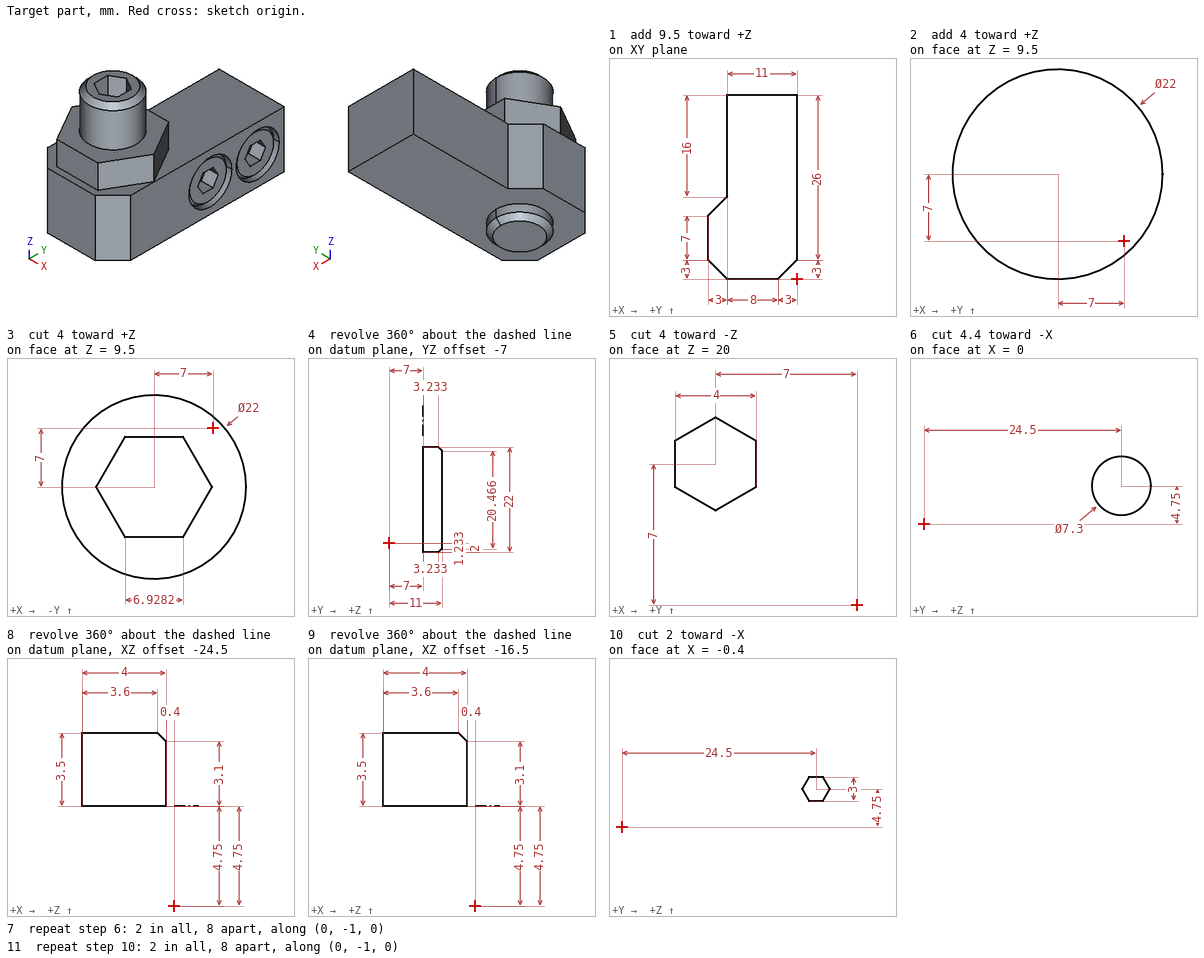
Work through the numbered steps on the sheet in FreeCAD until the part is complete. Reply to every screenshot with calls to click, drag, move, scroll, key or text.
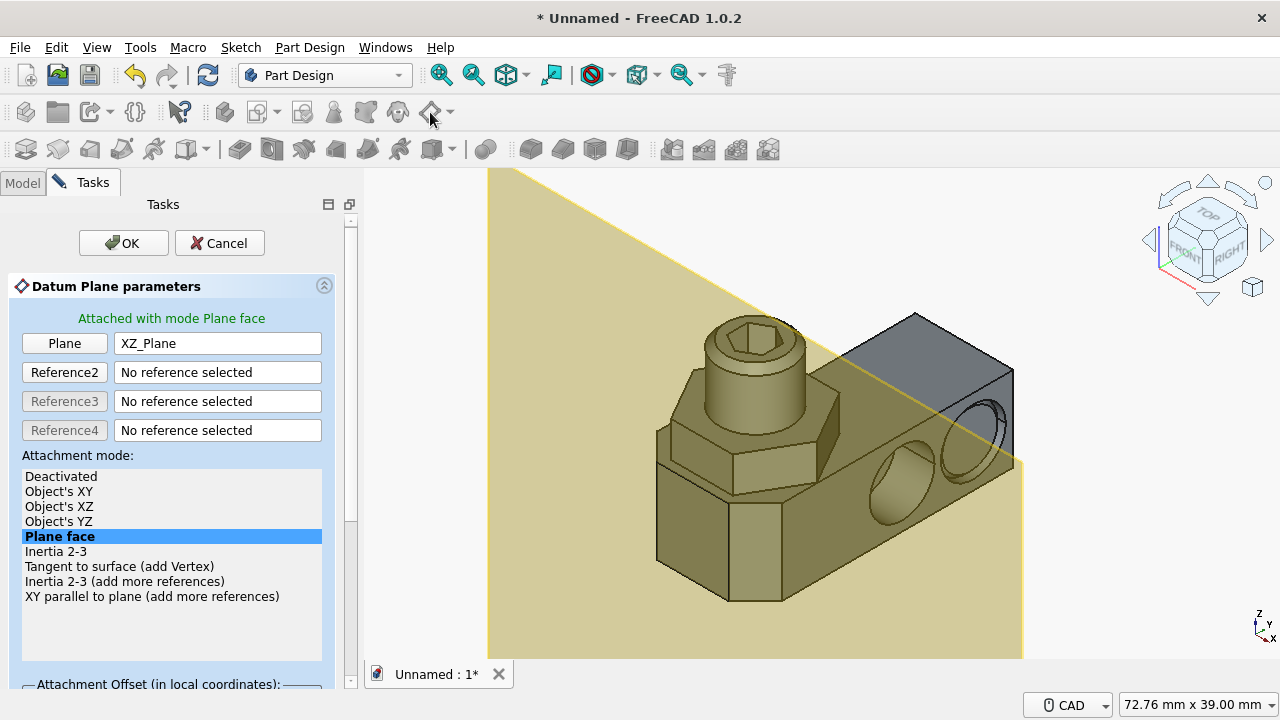
scroll(351, 451, down, 3)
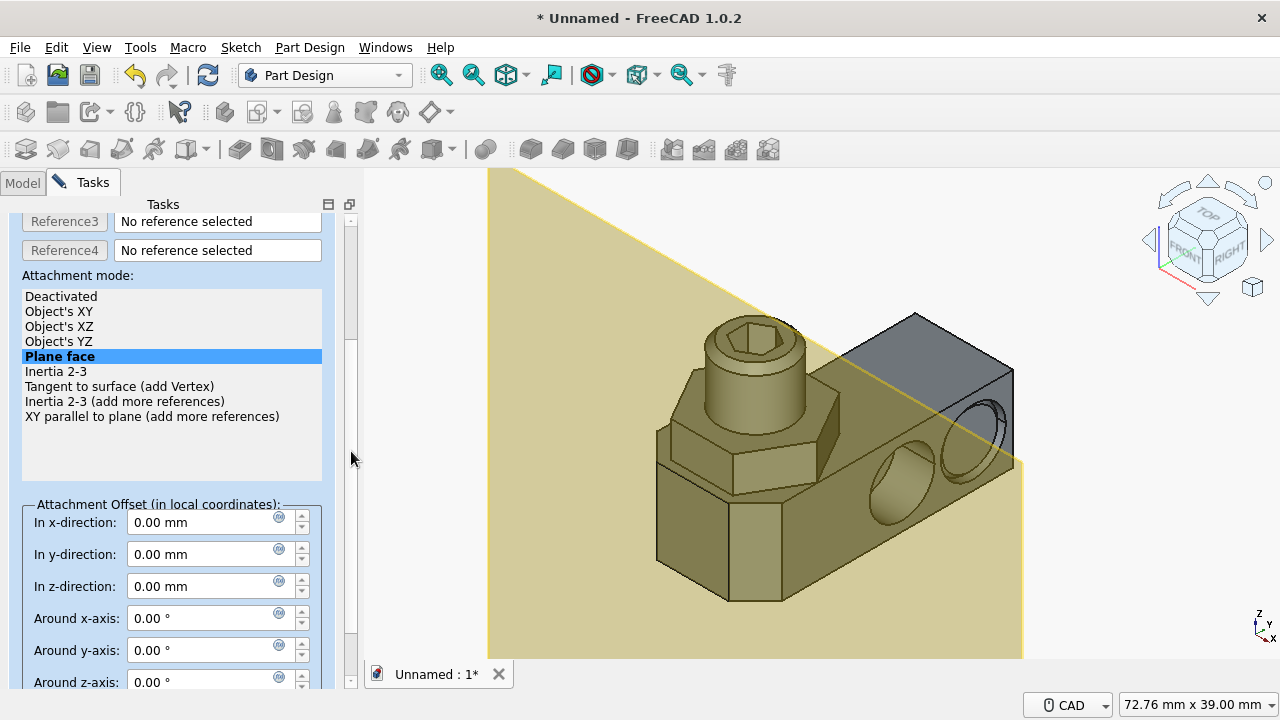
triple_click(210, 586)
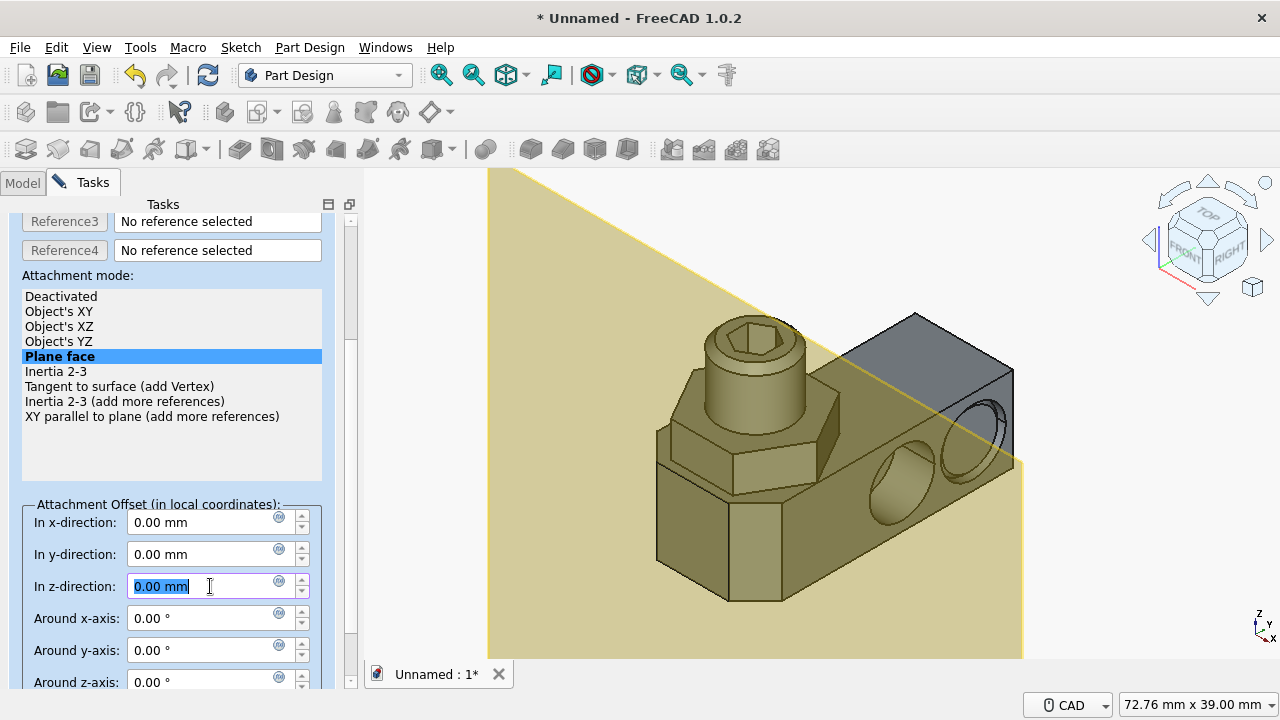
text(-16.5)
key(Tab)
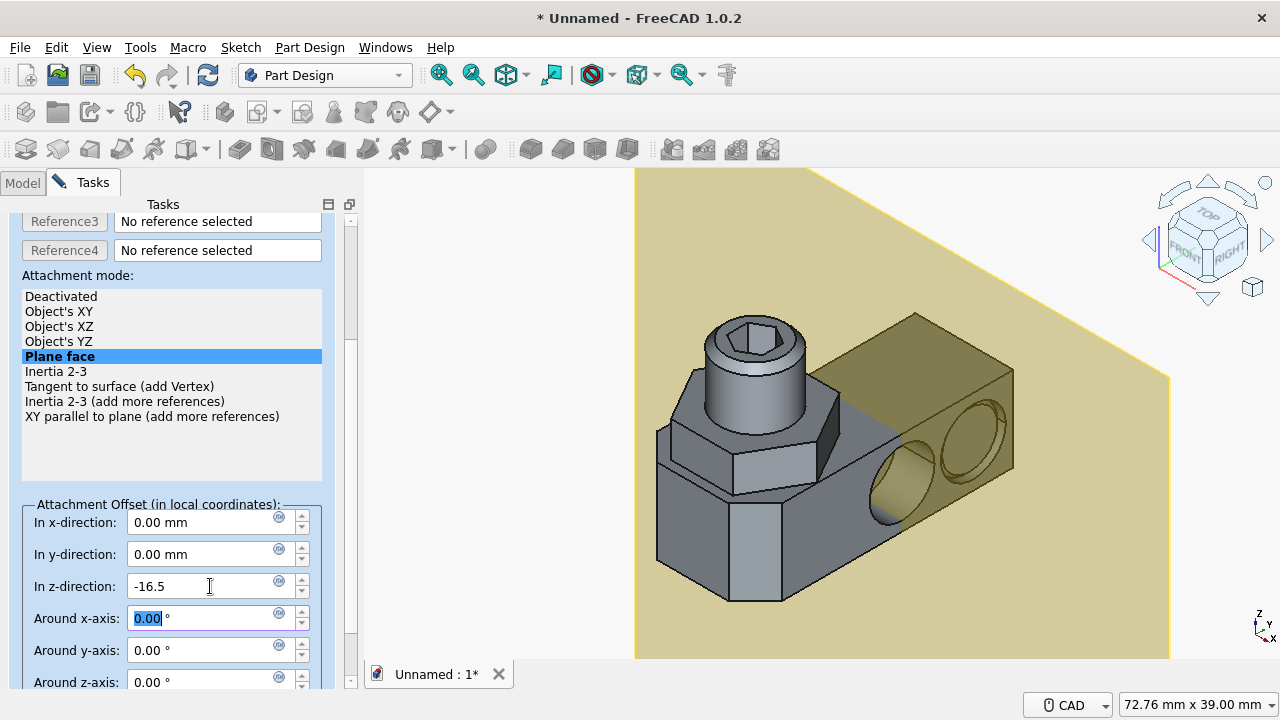
scroll(351, 451, up, 4)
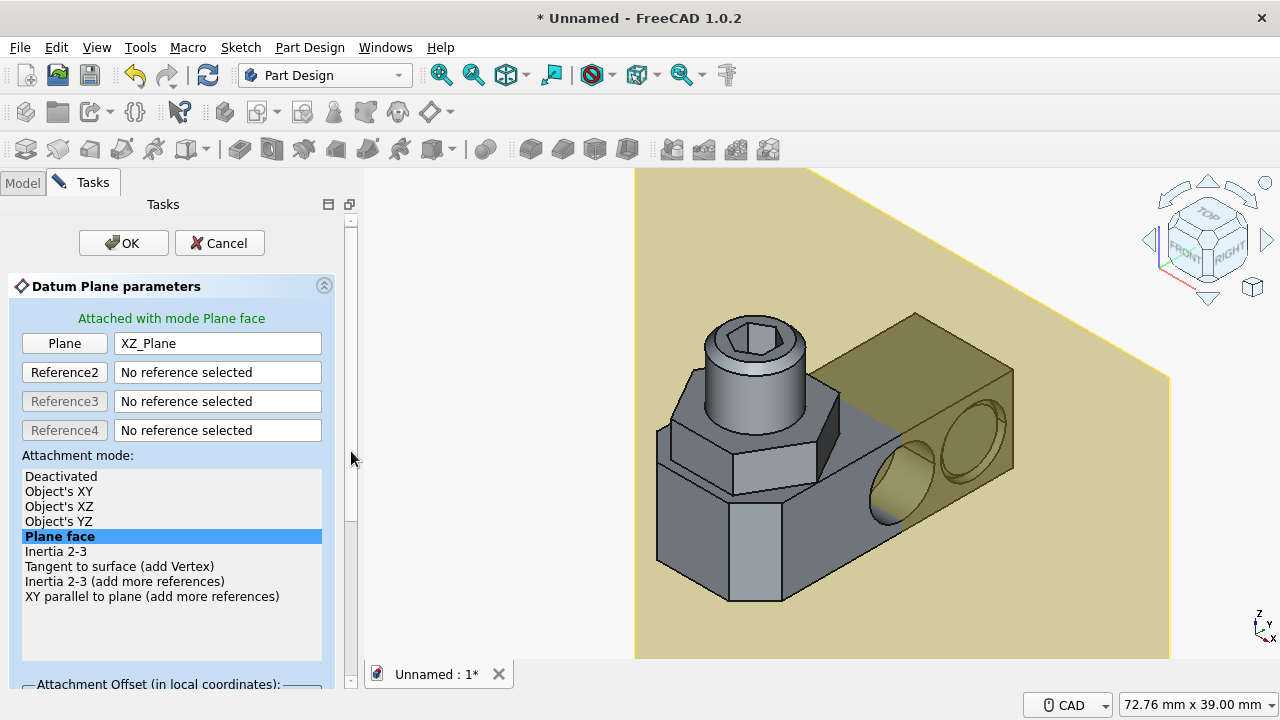
click(124, 243)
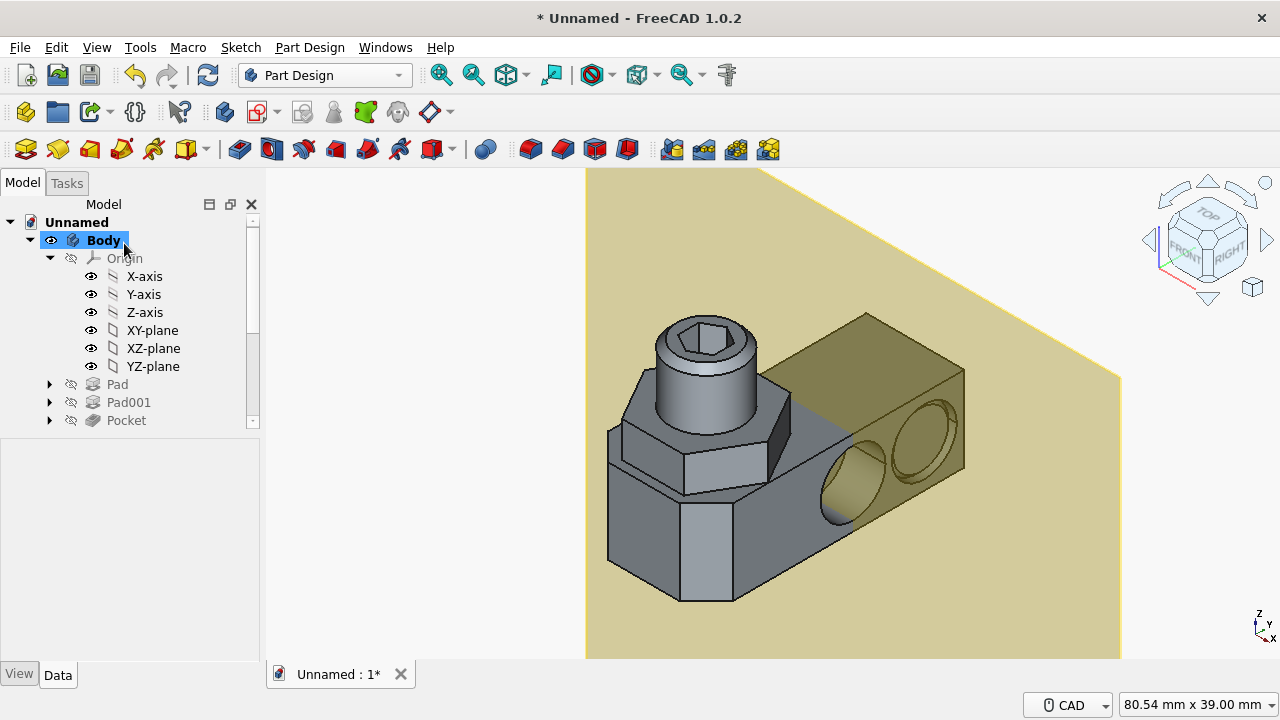
scroll(100, 326, down, 3)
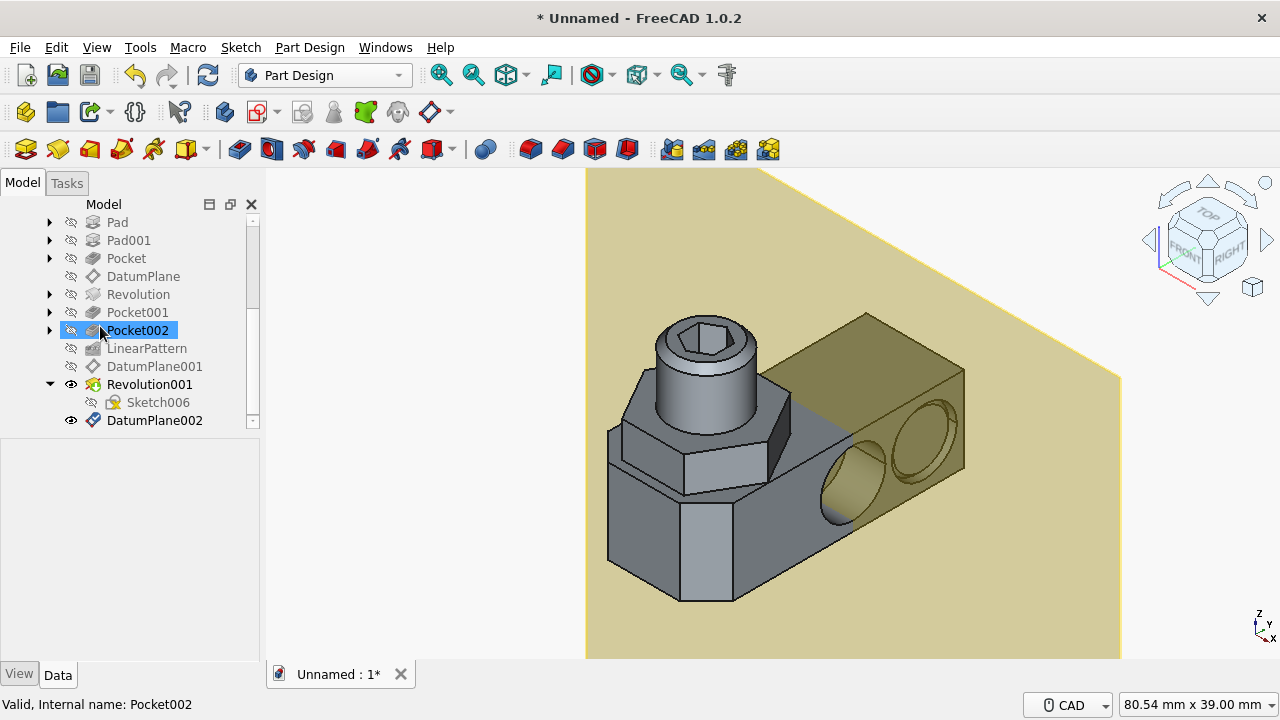
click(116, 420)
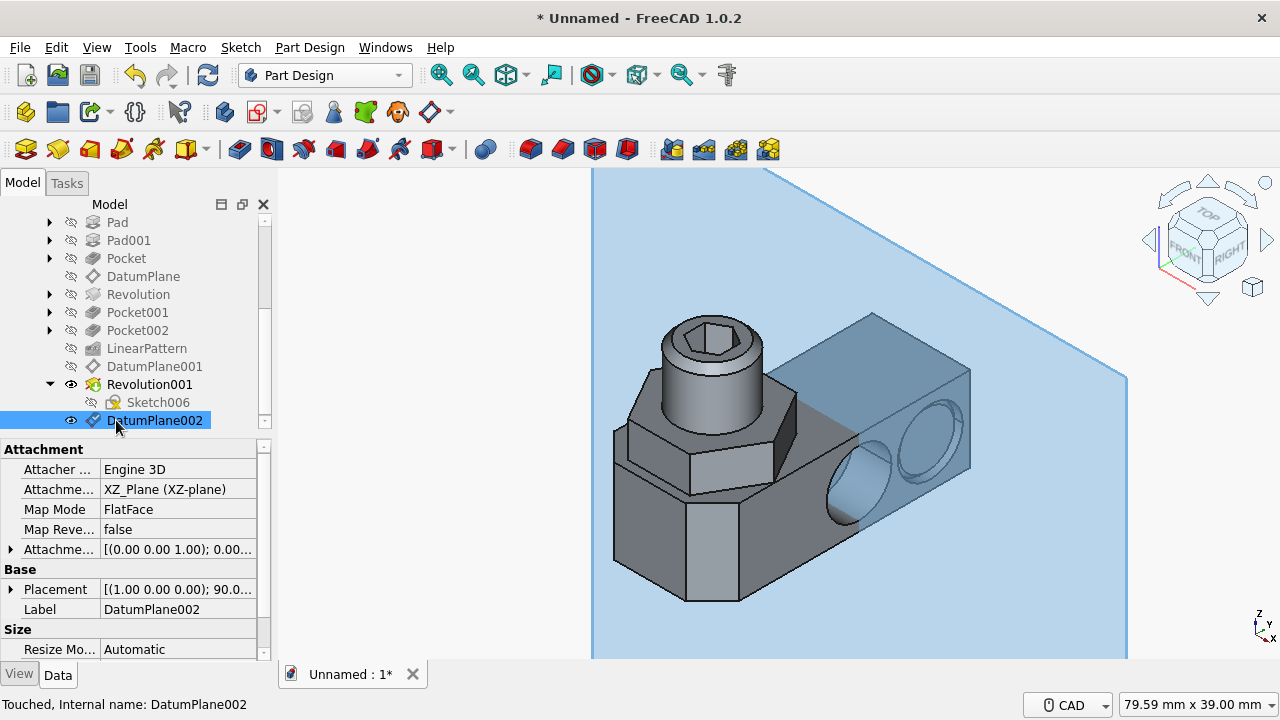
click(258, 112)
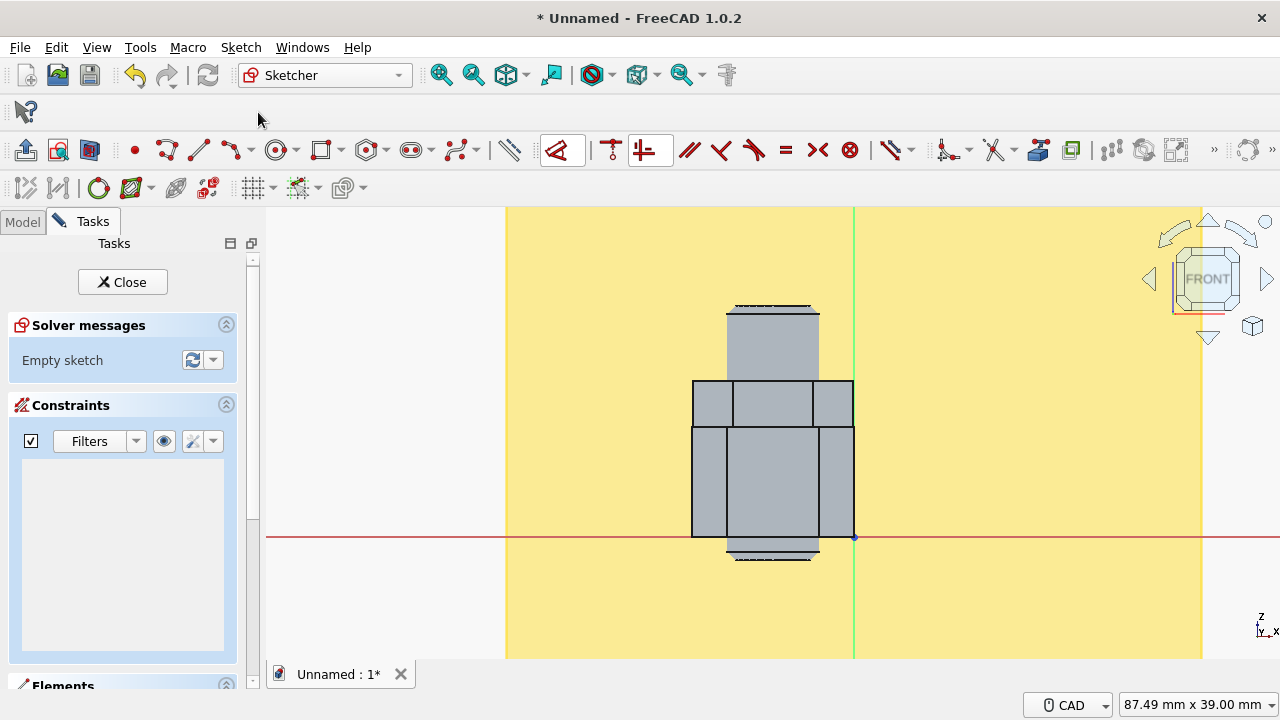
key(q)
key(s)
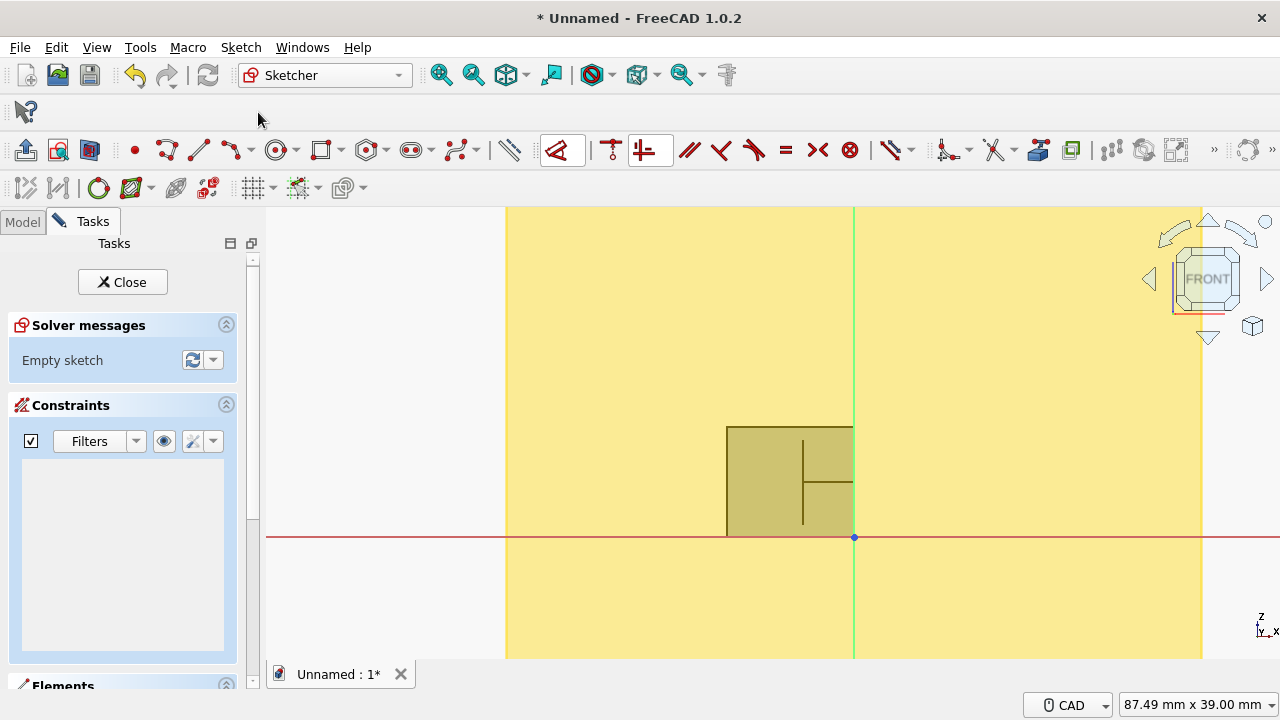
scroll(912, 522, up, 5)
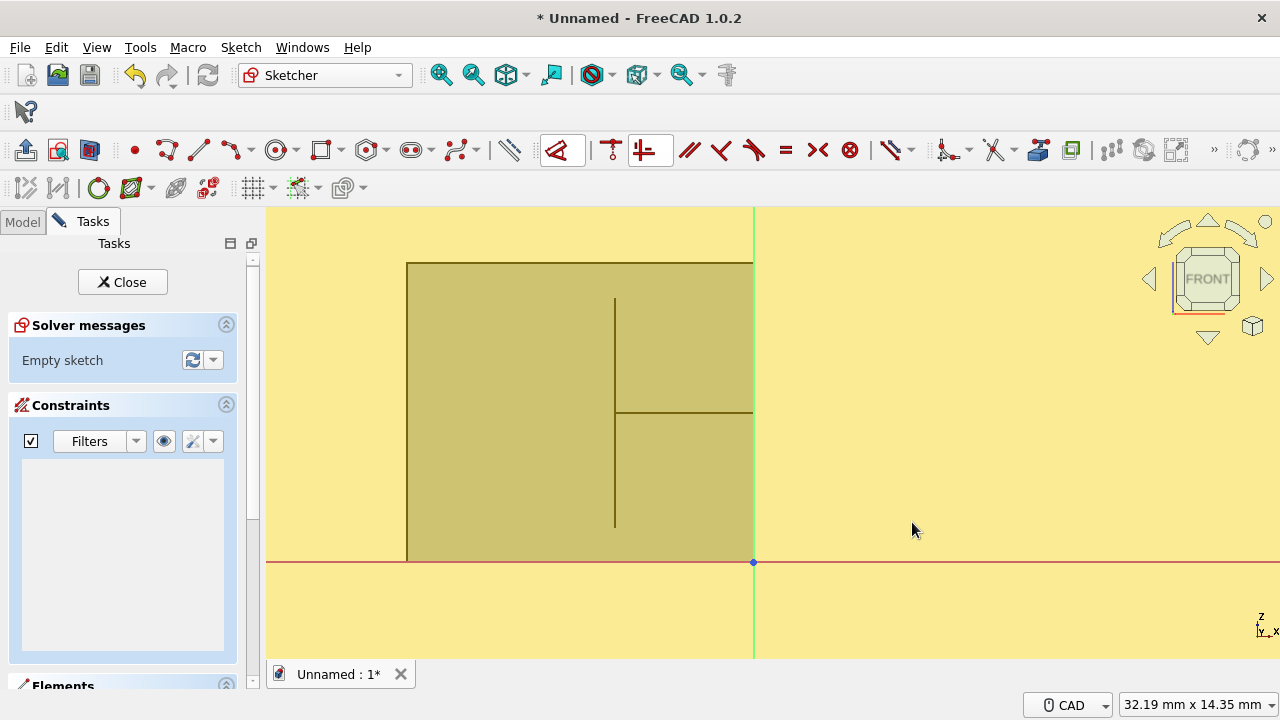
key(g)
key(m)